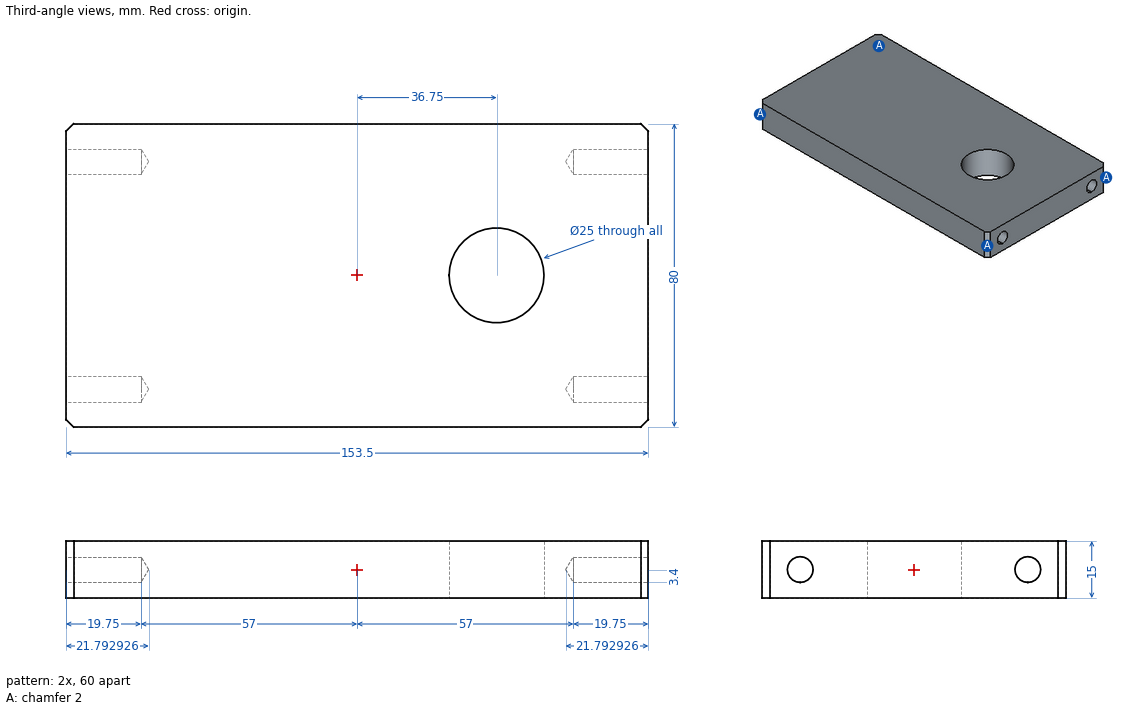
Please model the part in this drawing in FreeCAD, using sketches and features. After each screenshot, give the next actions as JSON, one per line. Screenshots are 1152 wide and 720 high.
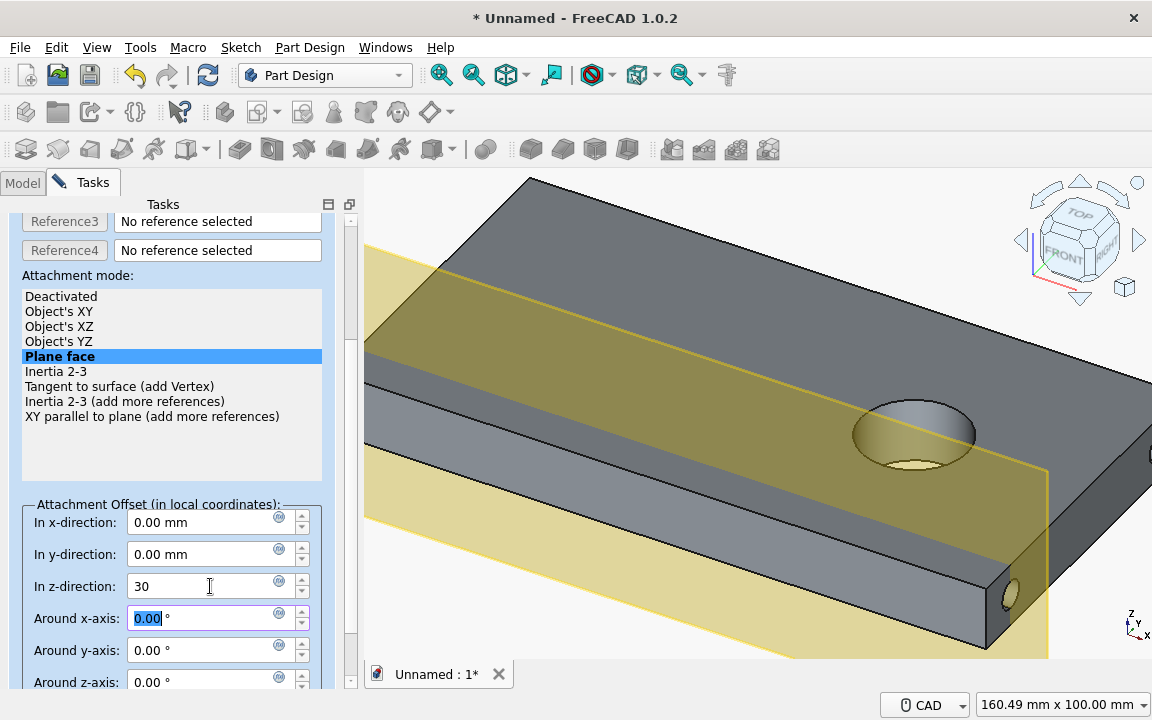
{"action": "scroll", "coordinate": [351, 451], "scroll_direction": "up", "scroll_amount": 4}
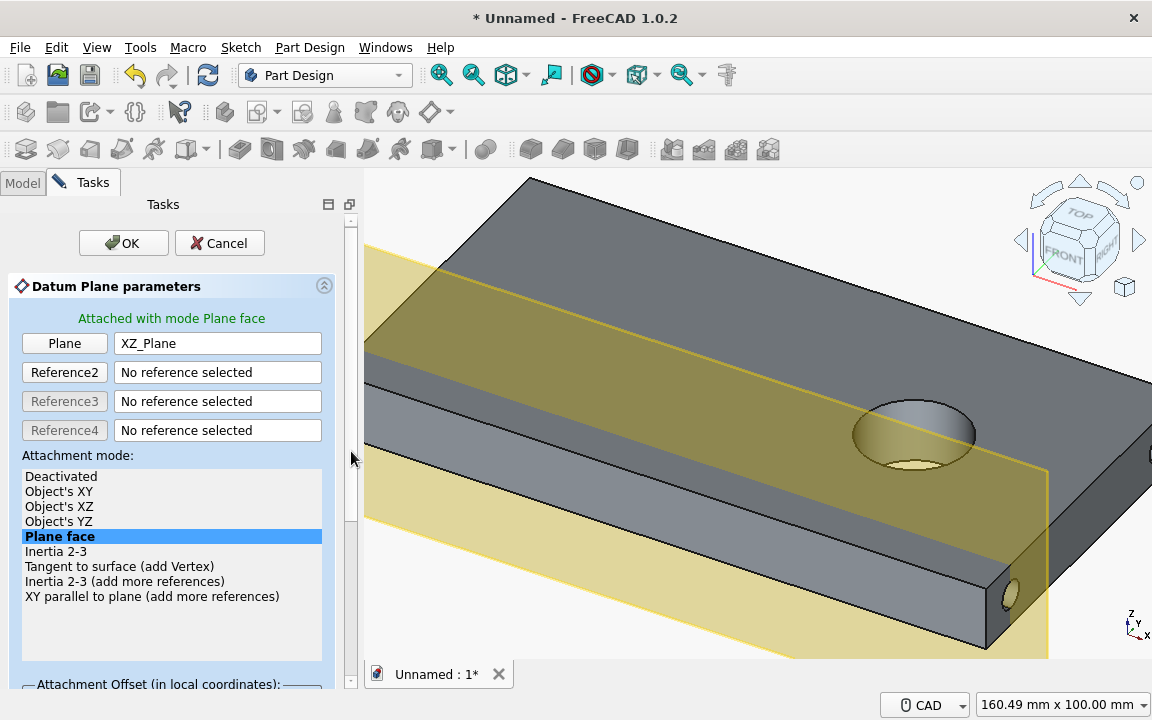
{"action": "left_click", "coordinate": [124, 243]}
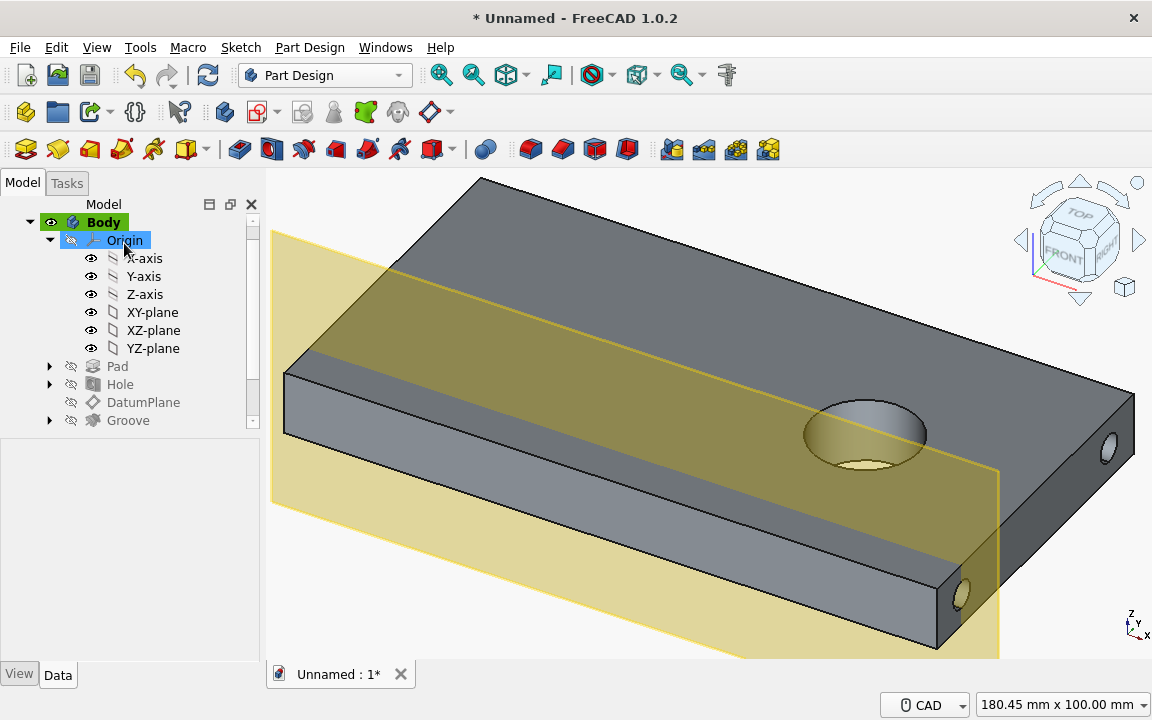
{"action": "scroll", "coordinate": [120, 326], "scroll_direction": "down", "scroll_amount": 3}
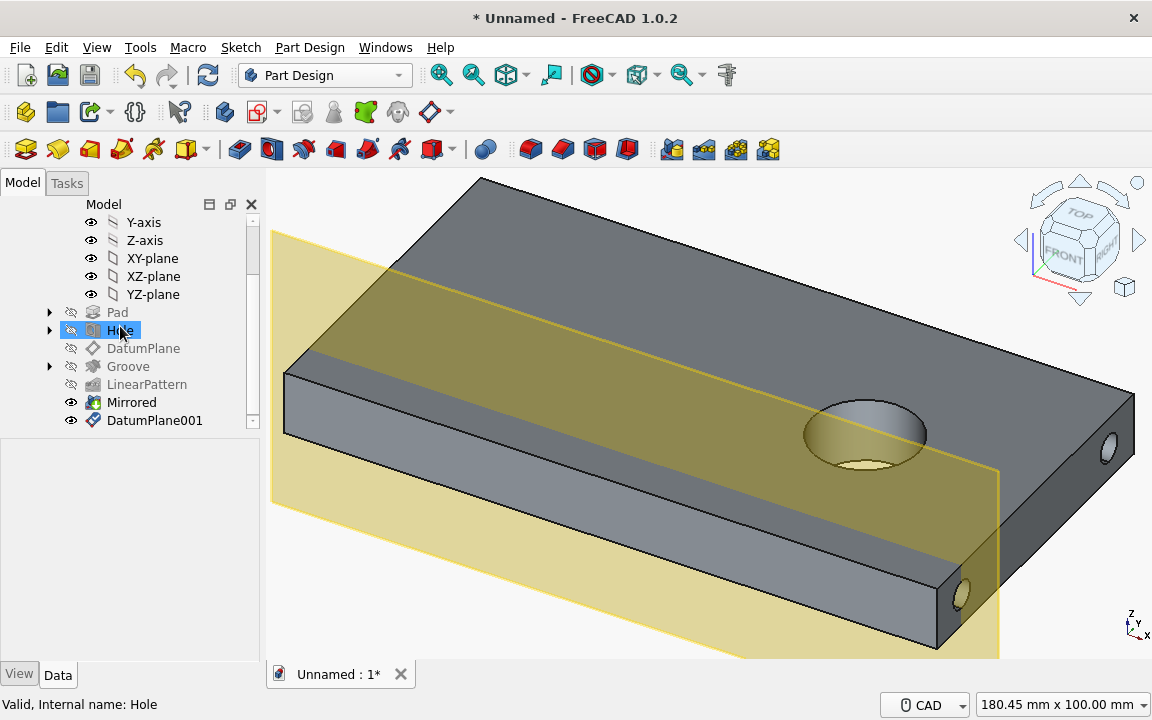
{"action": "left_click", "coordinate": [116, 420]}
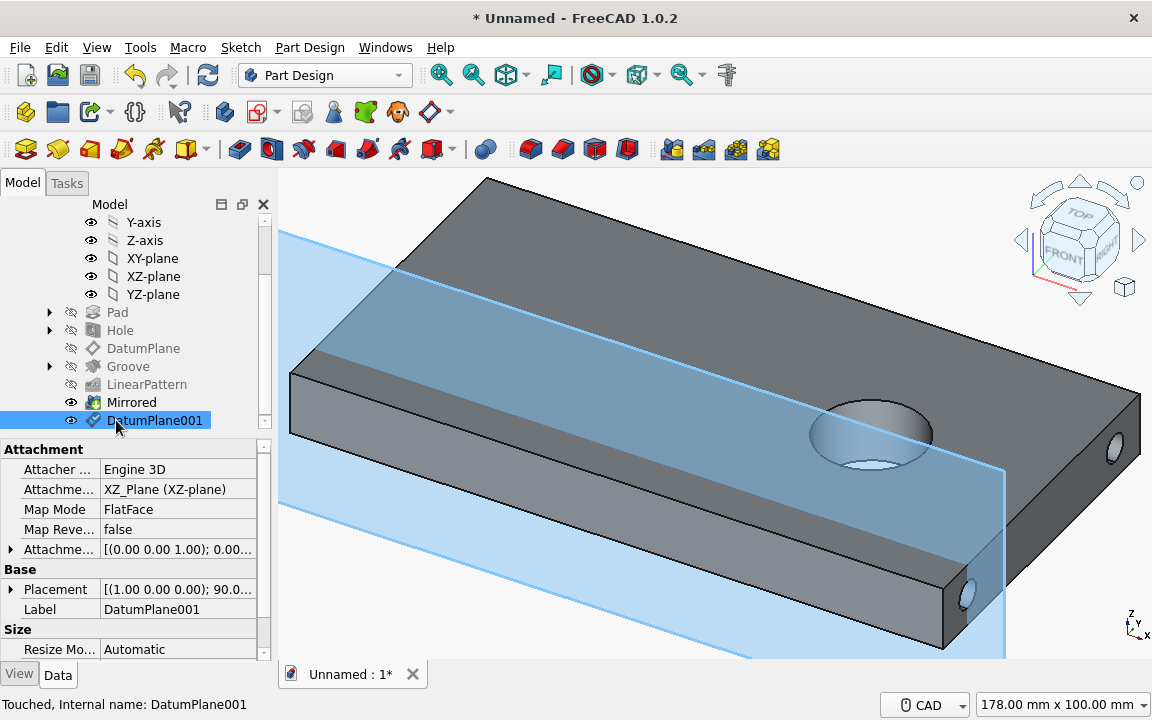
{"action": "left_click", "coordinate": [258, 112]}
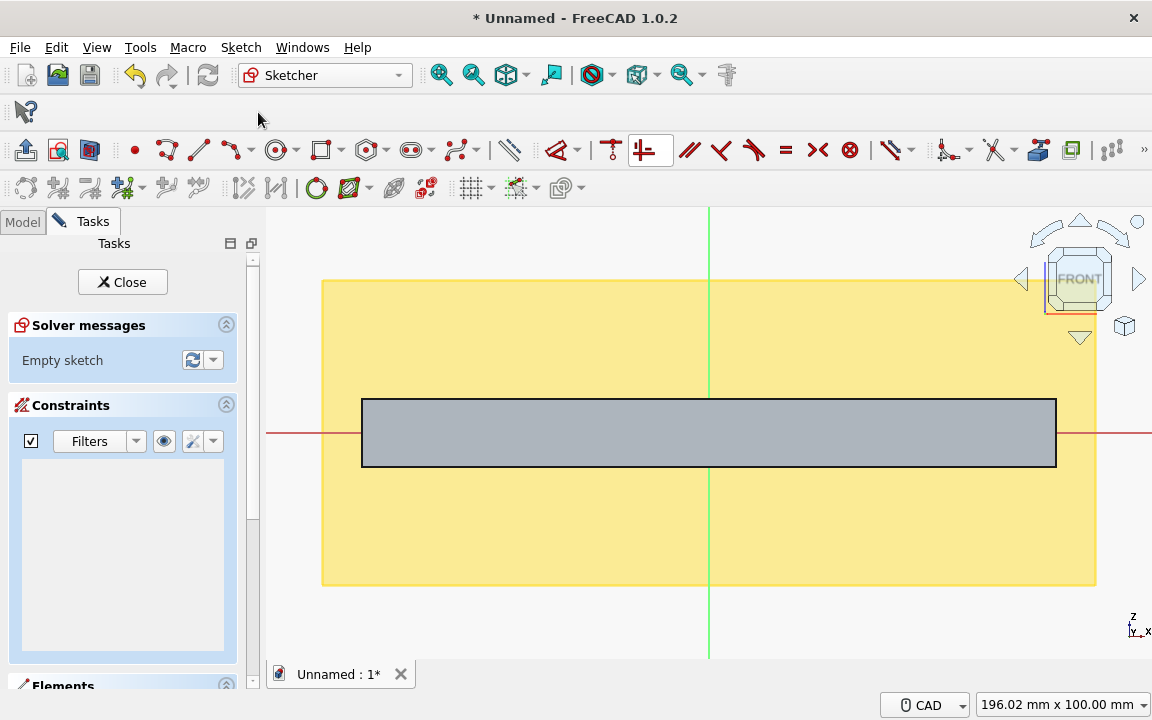
{"action": "key", "text": "q s"}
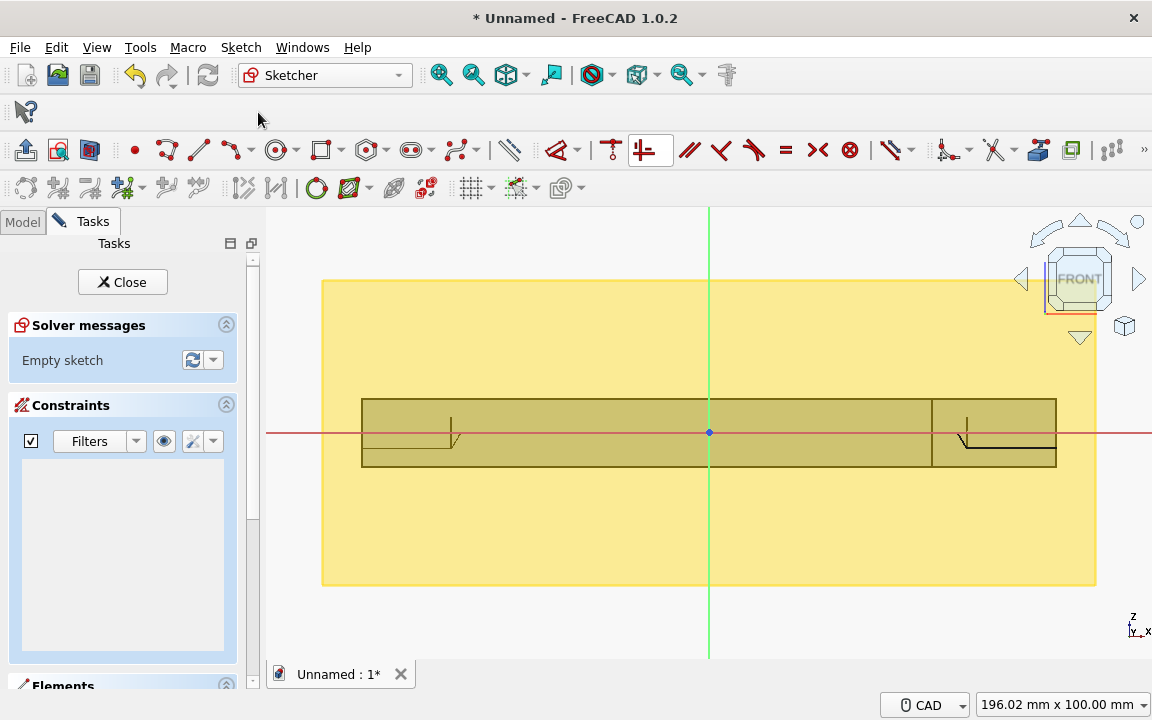
{"action": "scroll", "coordinate": [353, 443], "scroll_direction": "up", "scroll_amount": 8}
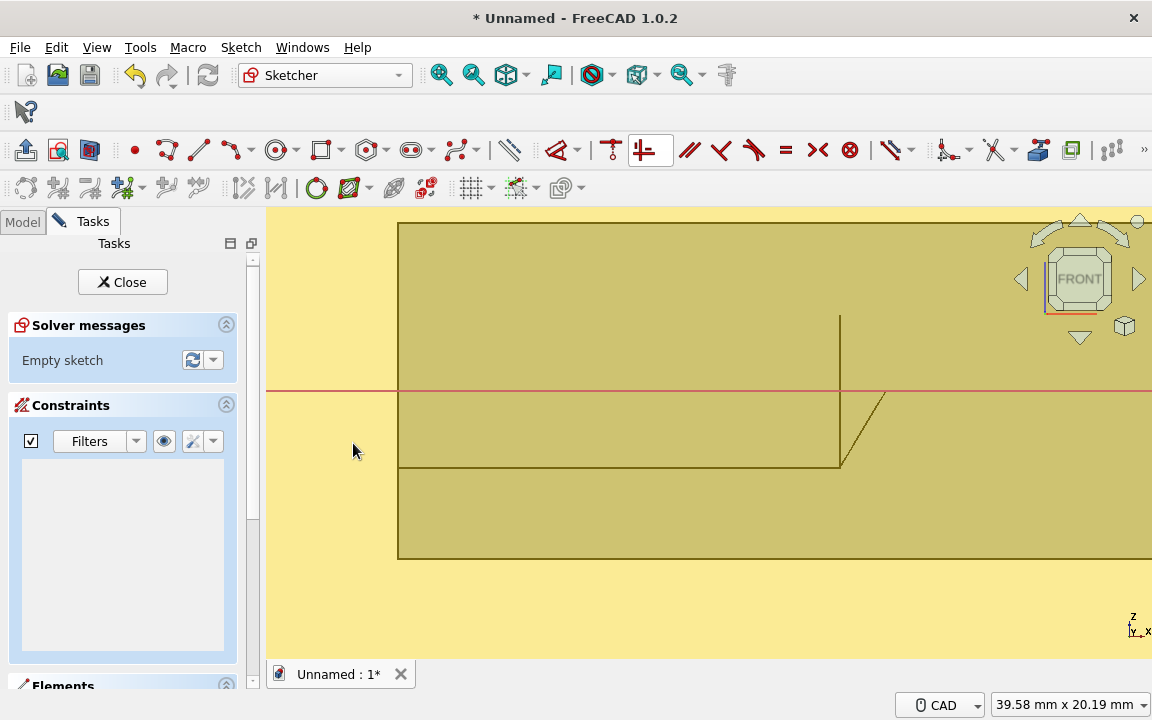
{"action": "left_click", "coordinate": [168, 150]}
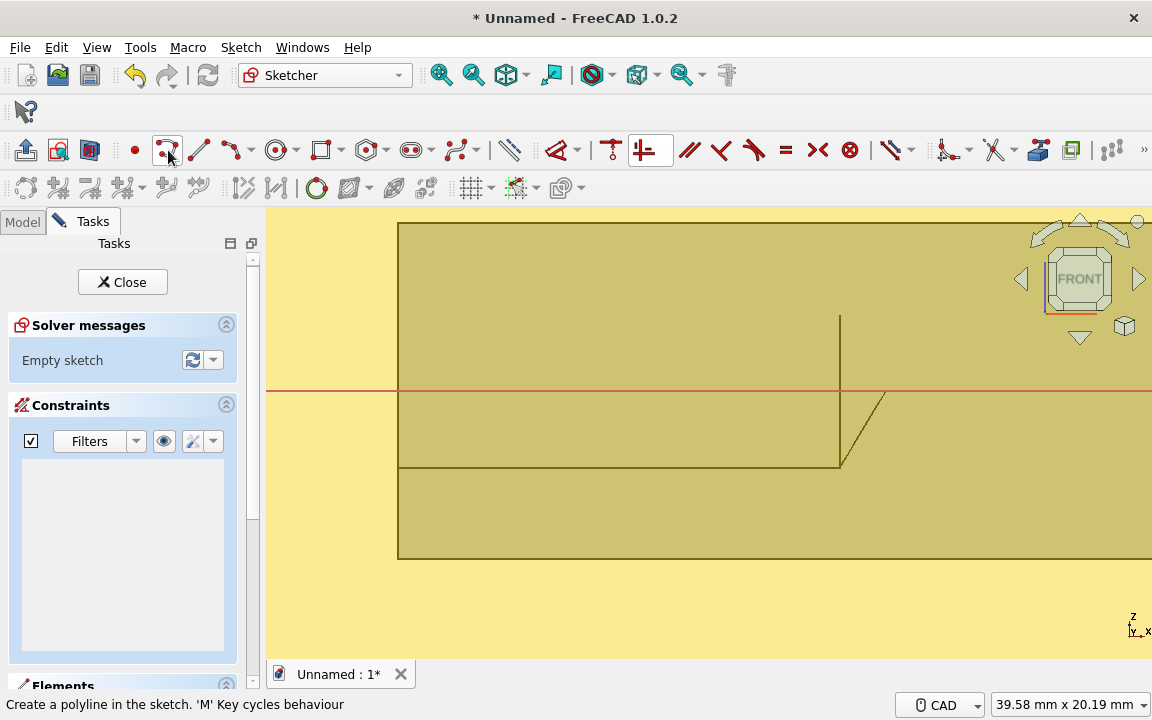
{"action": "left_click", "coordinate": [886, 391]}
{"action": "left_click", "coordinate": [840, 468]}
{"action": "left_click", "coordinate": [398, 468]}
{"action": "left_click", "coordinate": [398, 400]}
{"action": "left_click", "coordinate": [886, 391]}
{"action": "key", "text": "Escape"}
{"action": "key", "text": "Escape"}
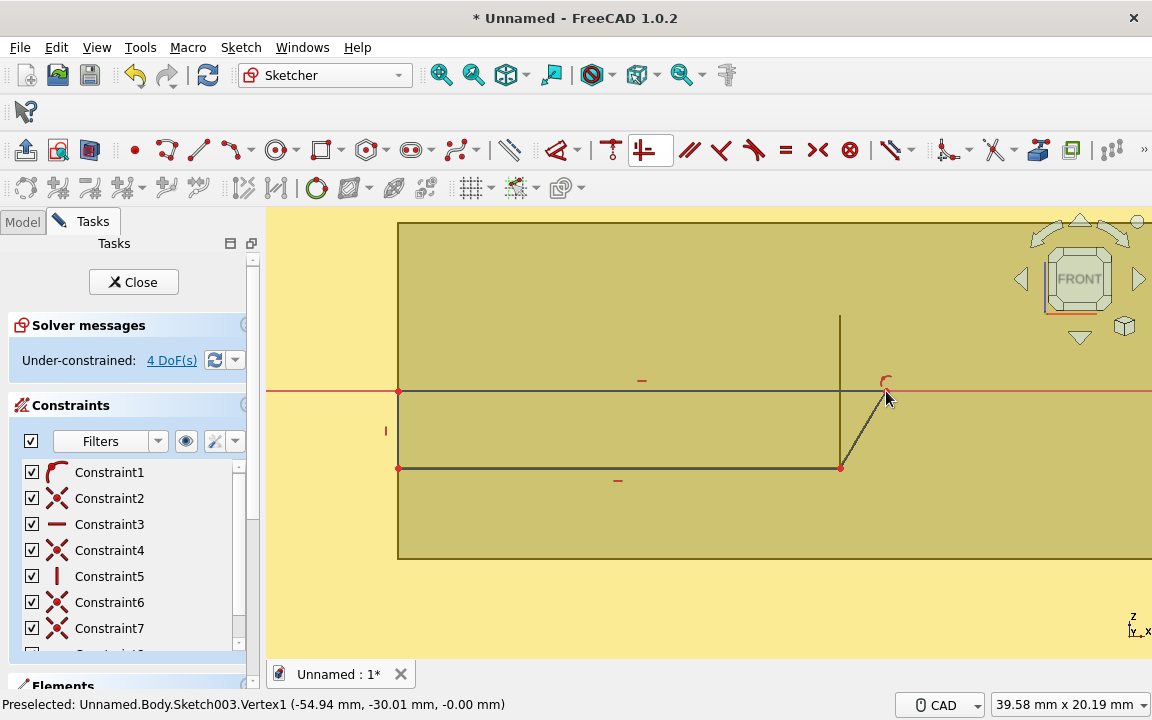
{"action": "left_click", "coordinate": [556, 150]}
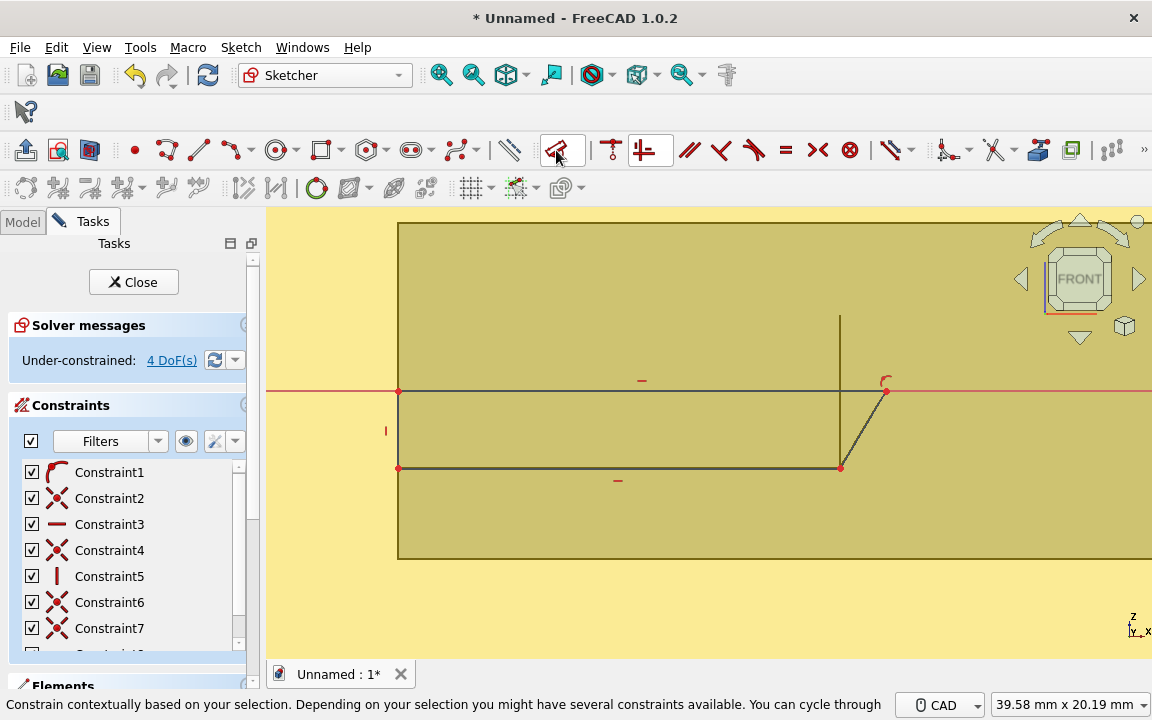
{"action": "left_click", "coordinate": [398, 446]}
{"action": "left_click", "coordinate": [364, 430]}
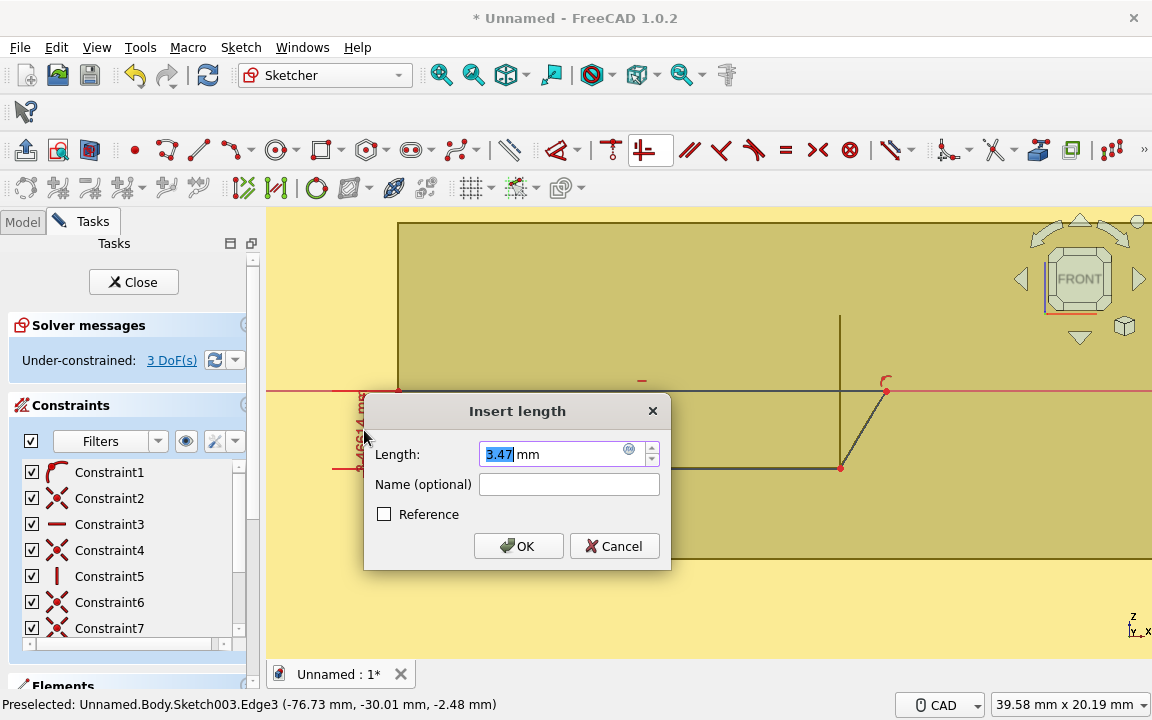
{"action": "type", "text": "3.4"}
{"action": "key", "text": "Return"}